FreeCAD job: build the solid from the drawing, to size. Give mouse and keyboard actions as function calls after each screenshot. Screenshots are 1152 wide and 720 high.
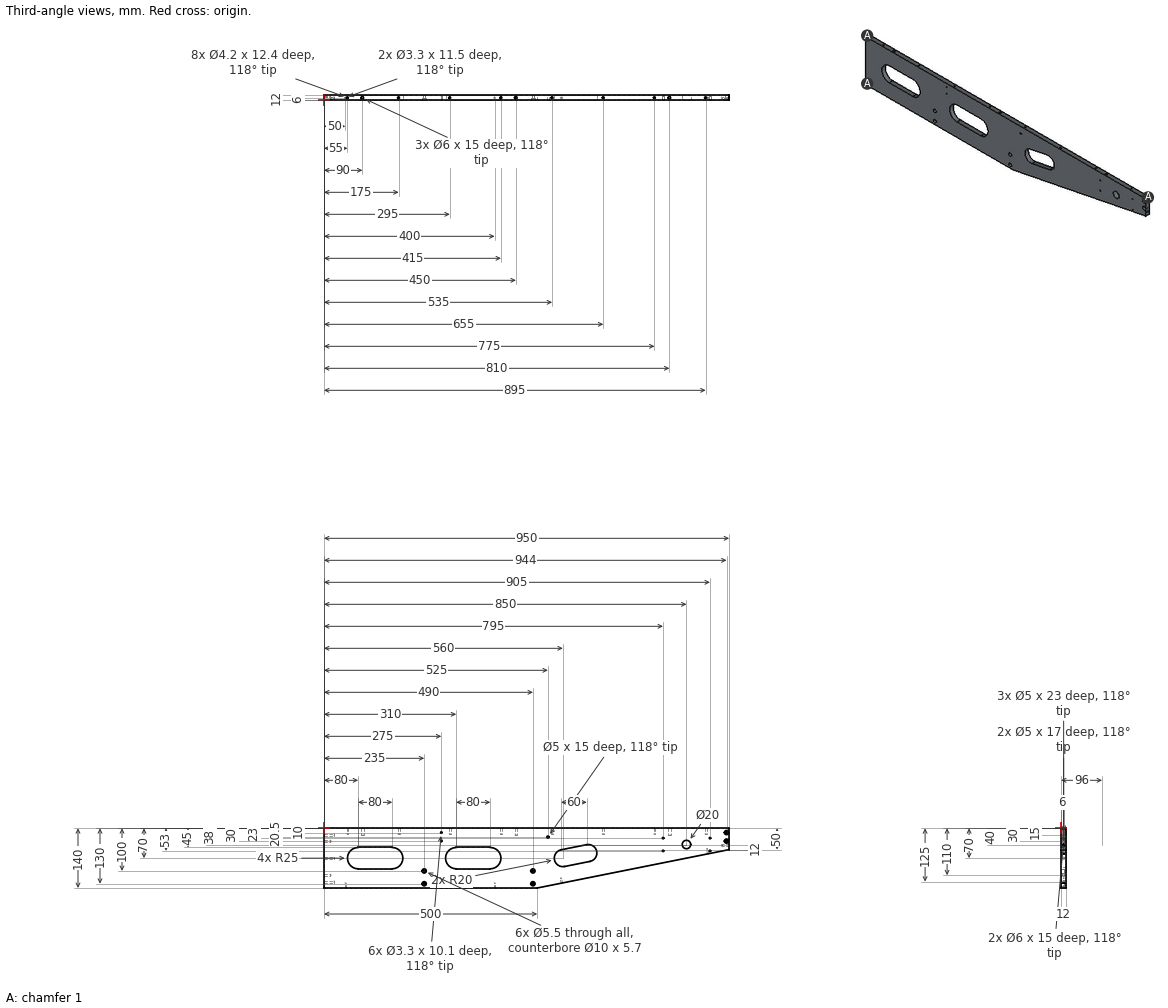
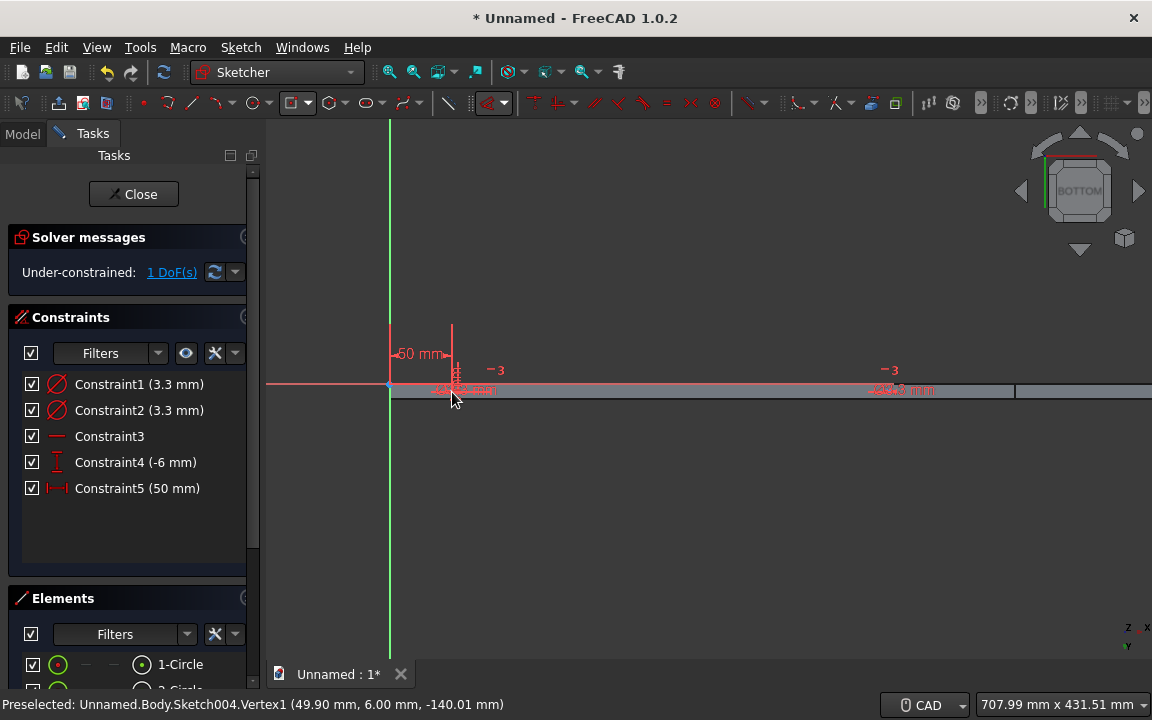
click(890, 392)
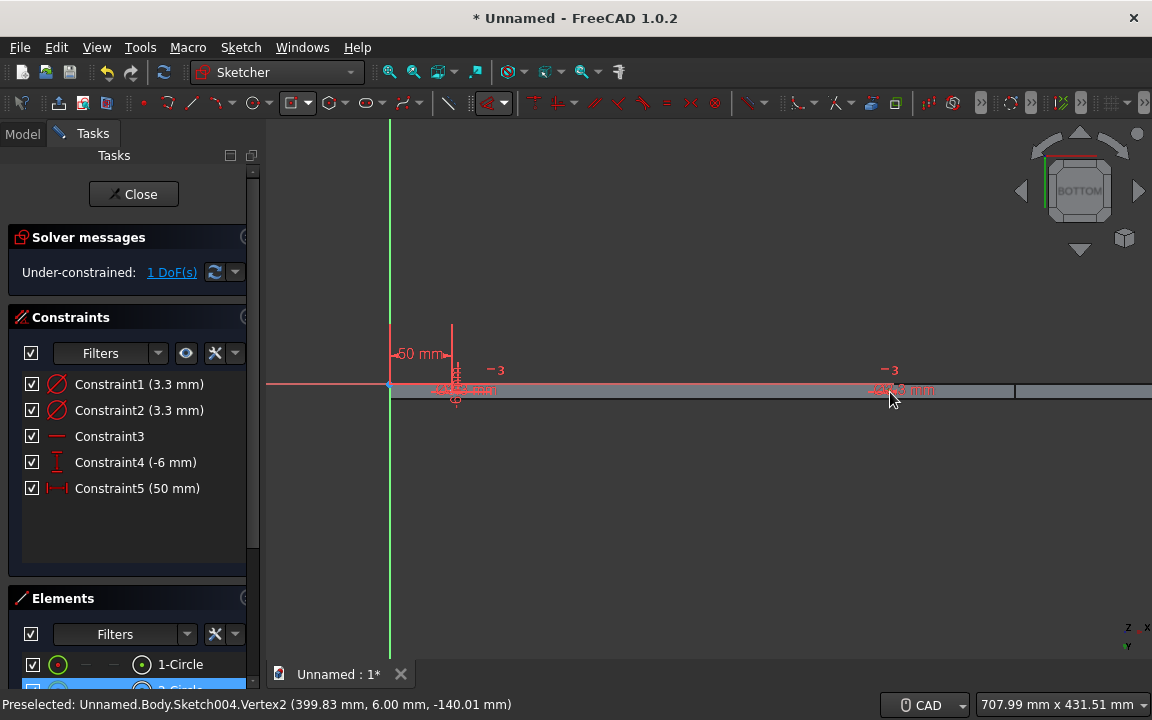
key(l)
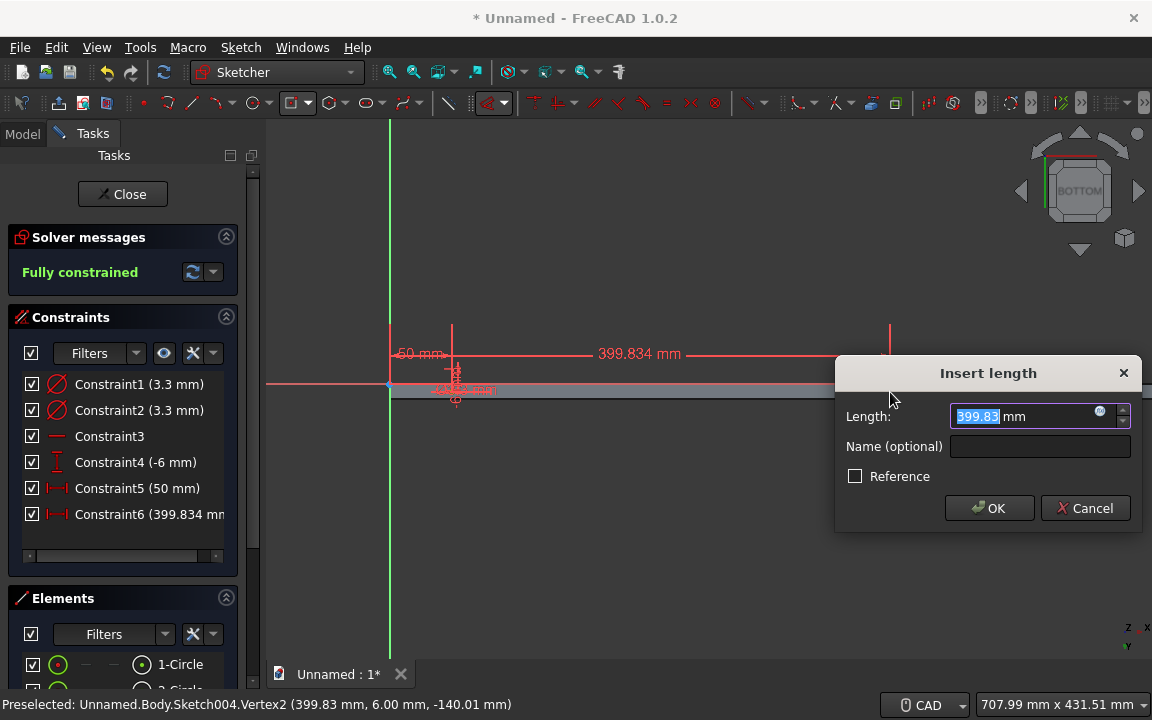
text(400)
key(Return)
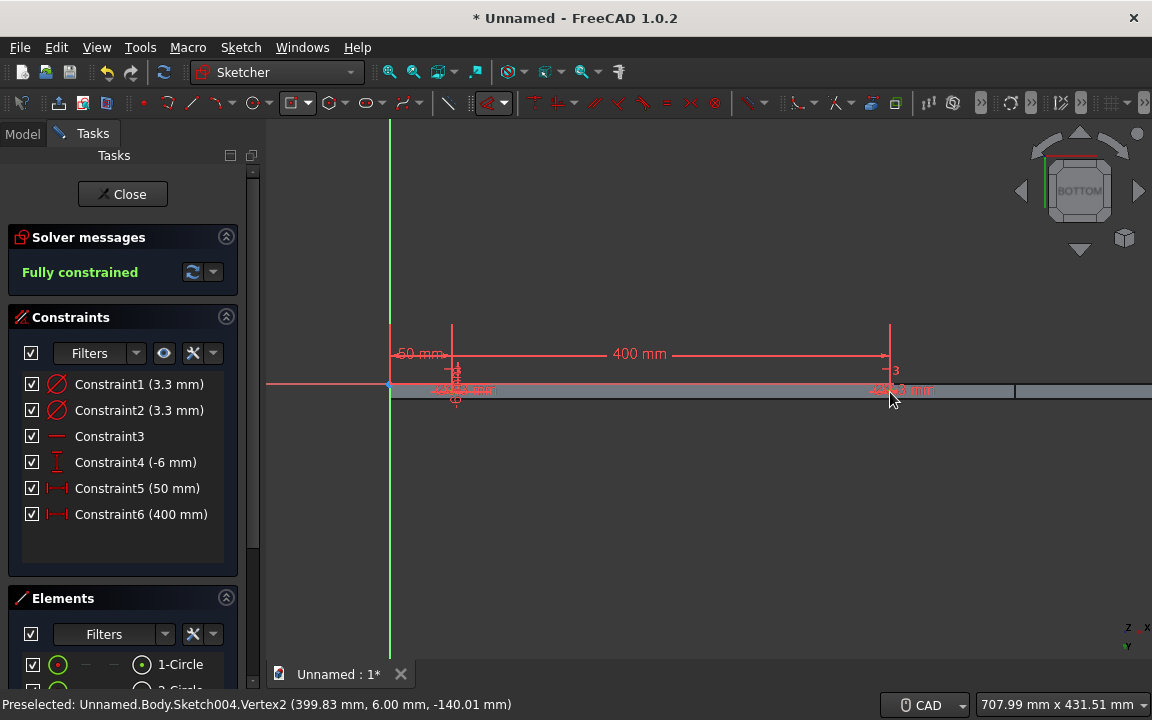
click(123, 194)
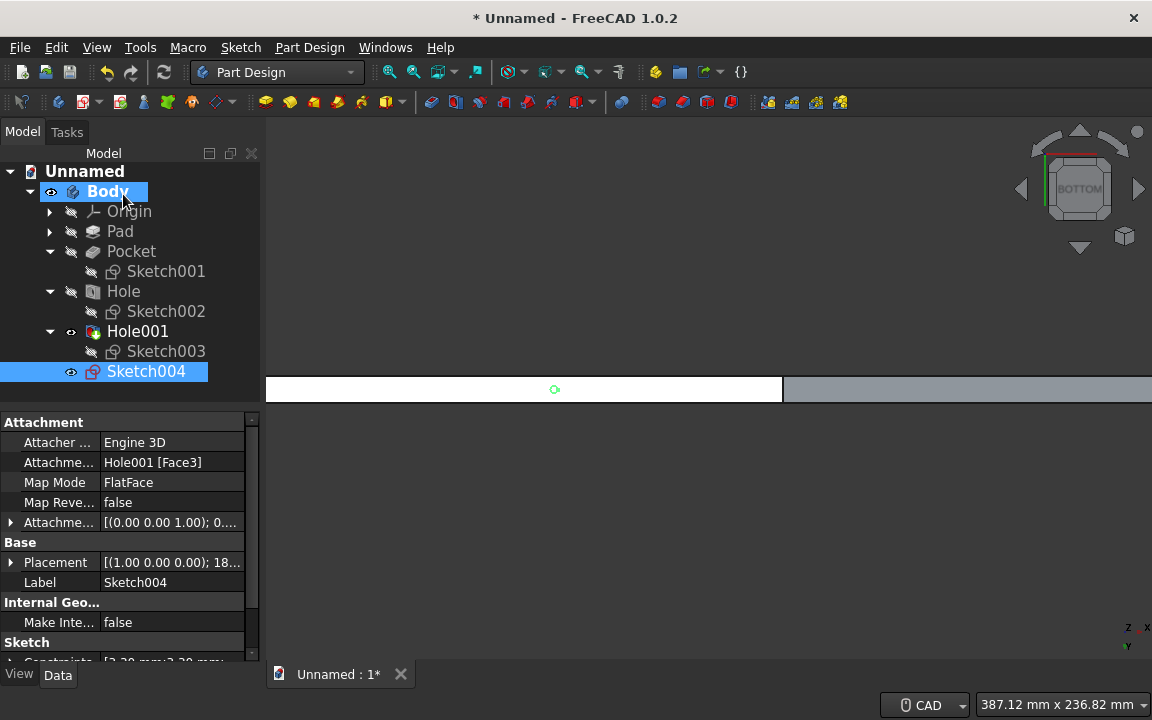
click(456, 102)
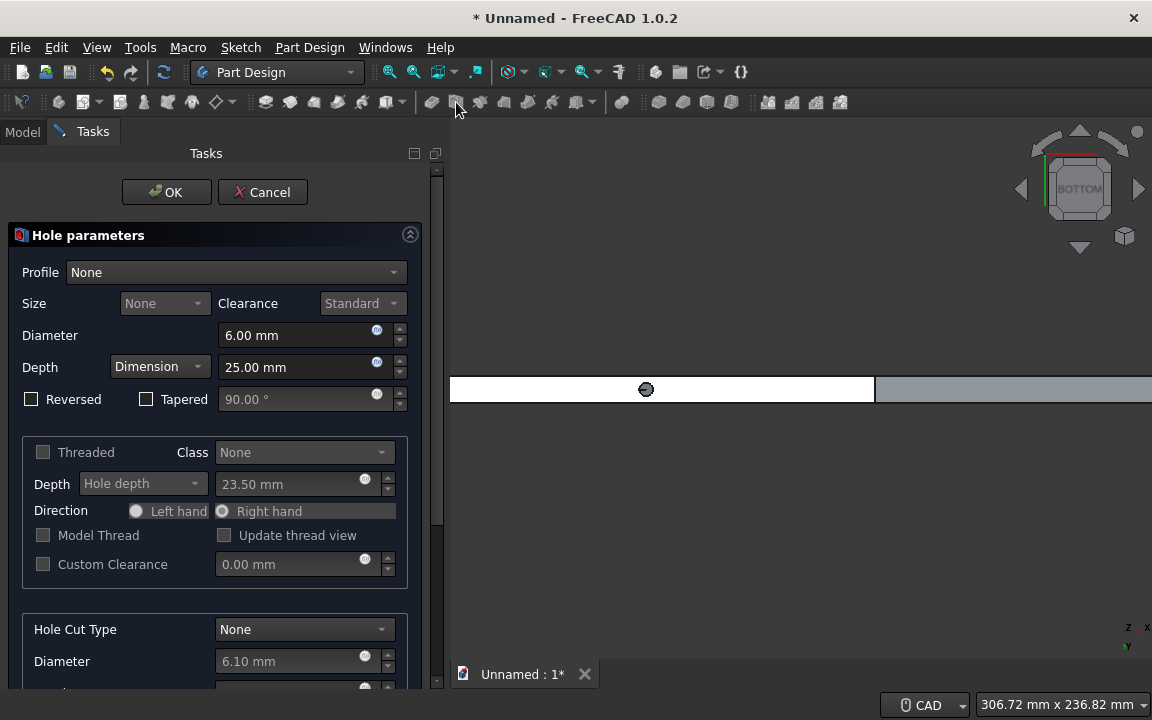
triple_click(305, 335)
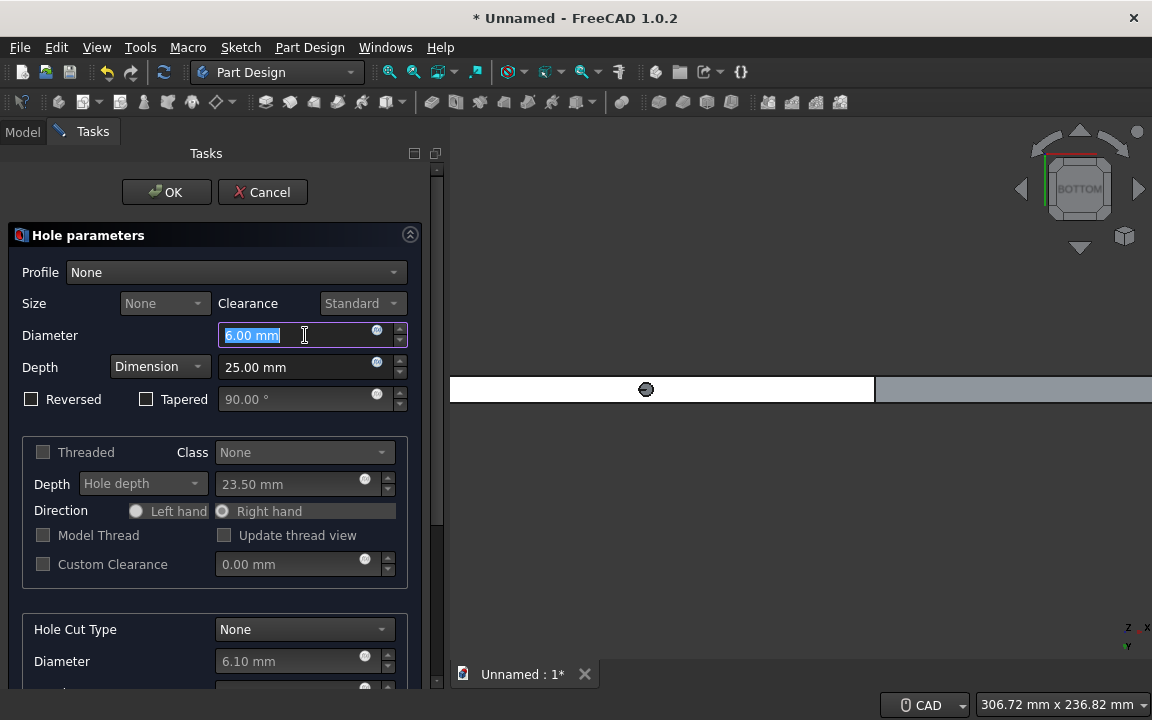
text(3.3)
key(Tab)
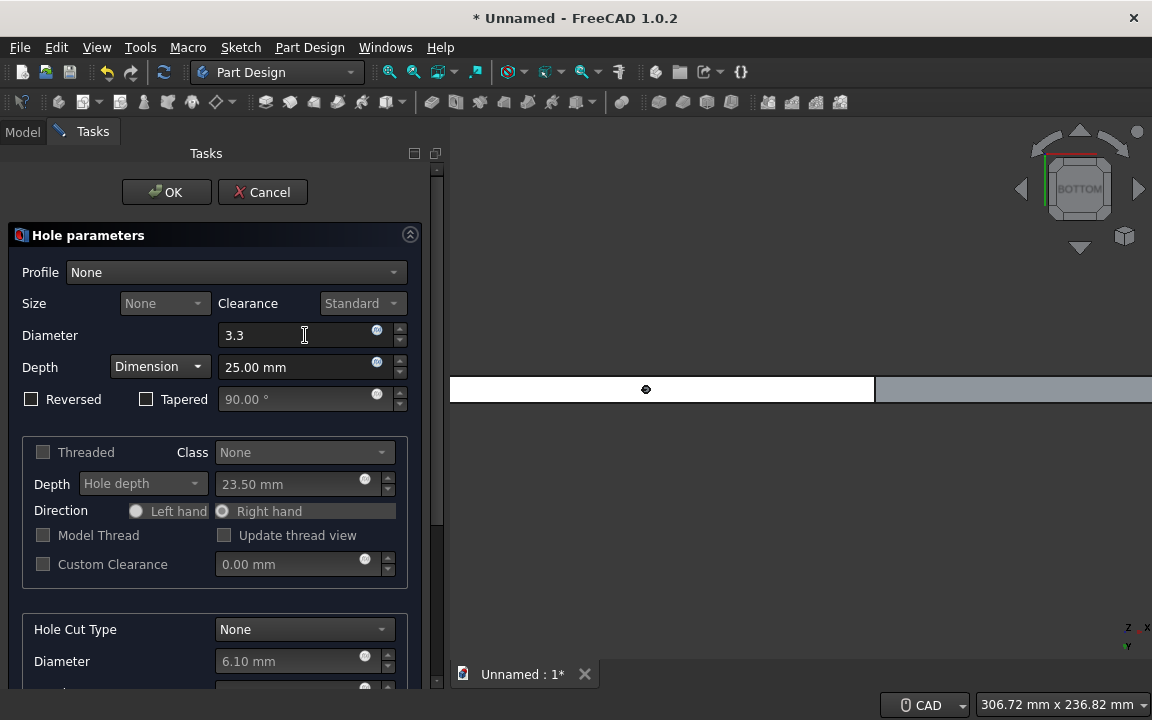
triple_click(305, 367)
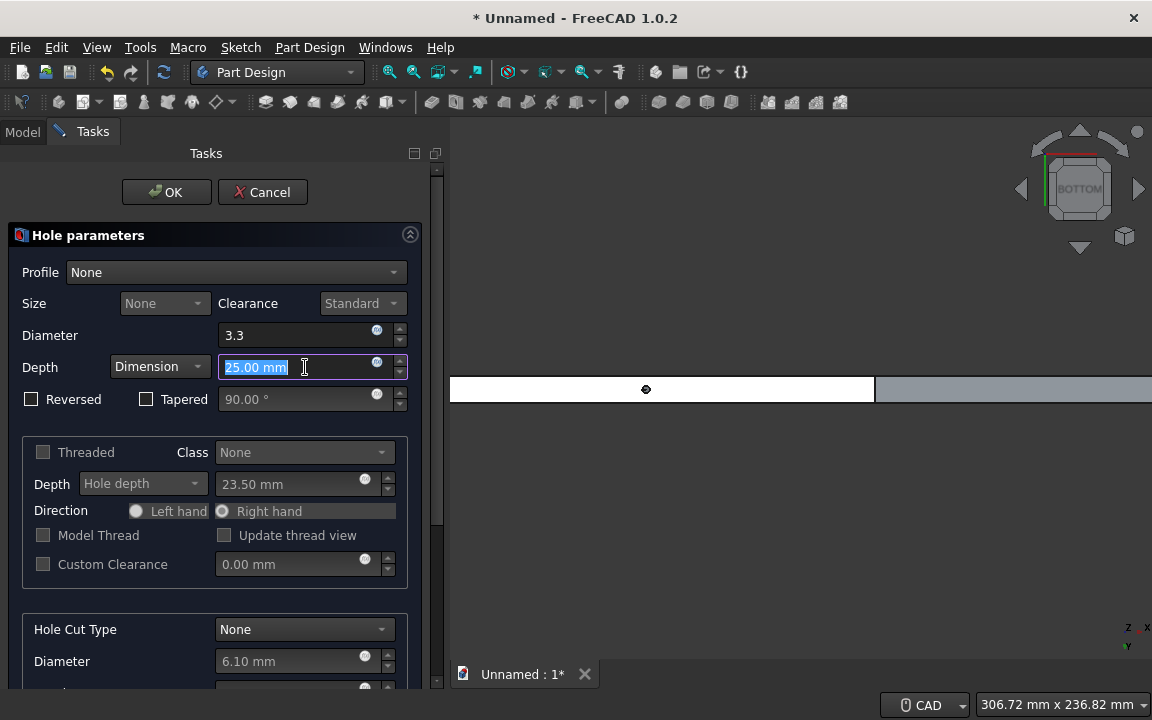
text(11.5)
key(Tab)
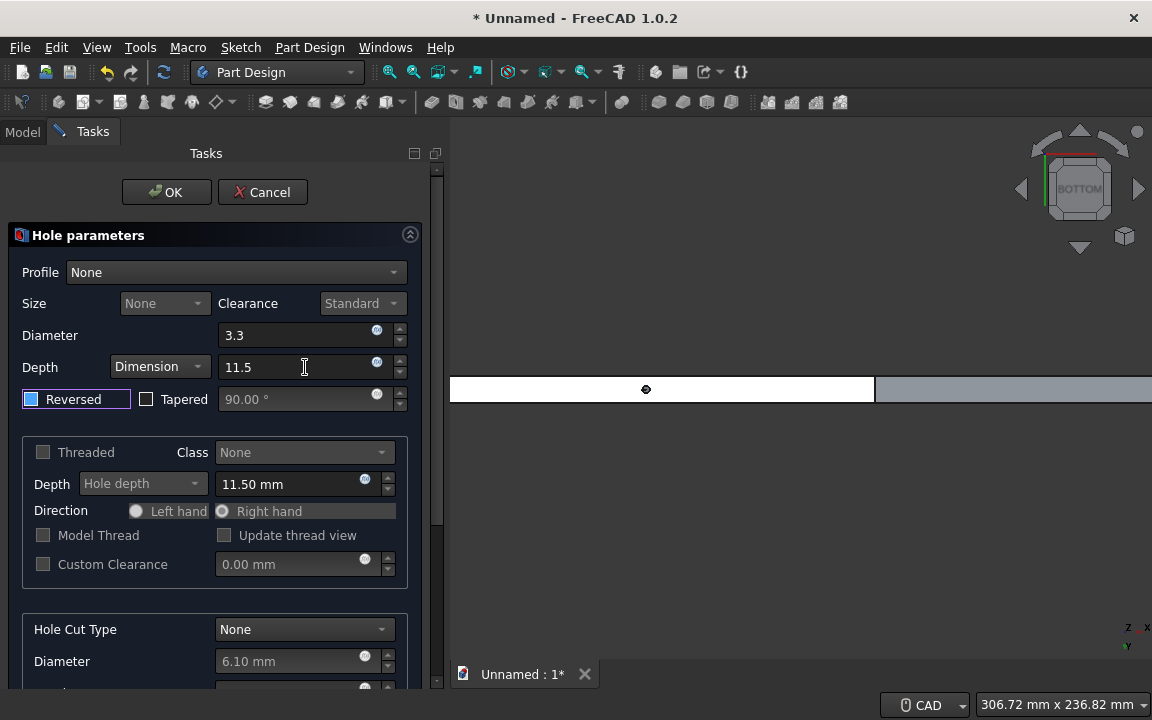
click(167, 192)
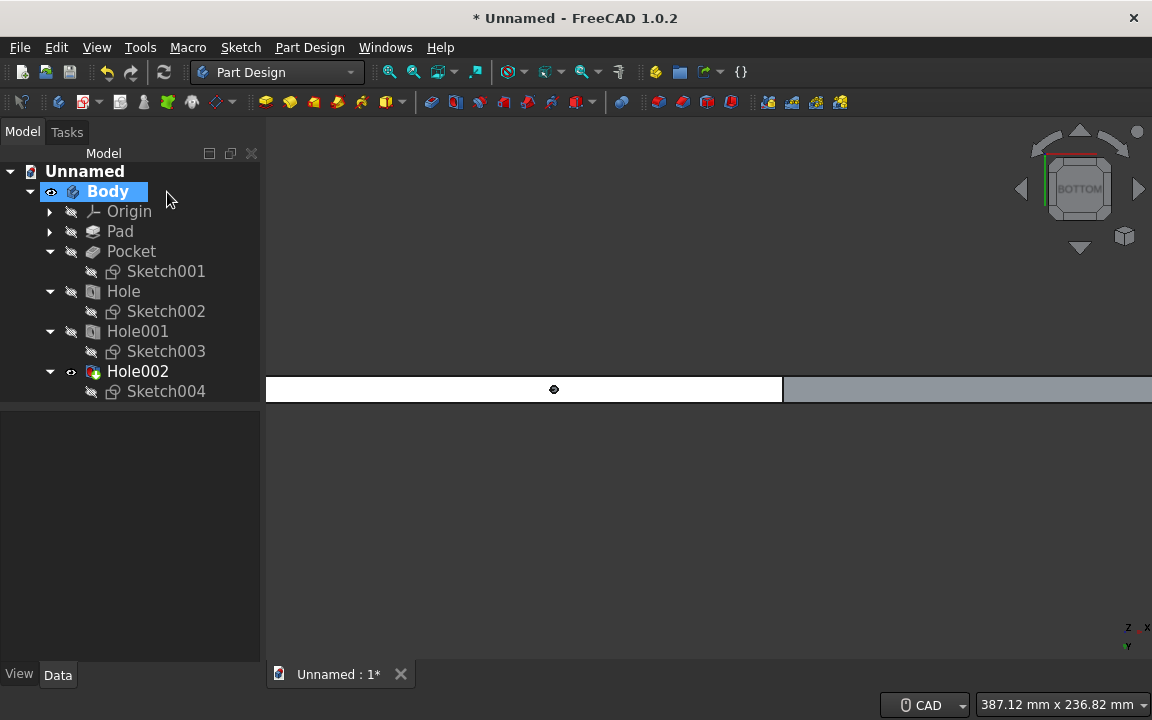
key(v)
key(f)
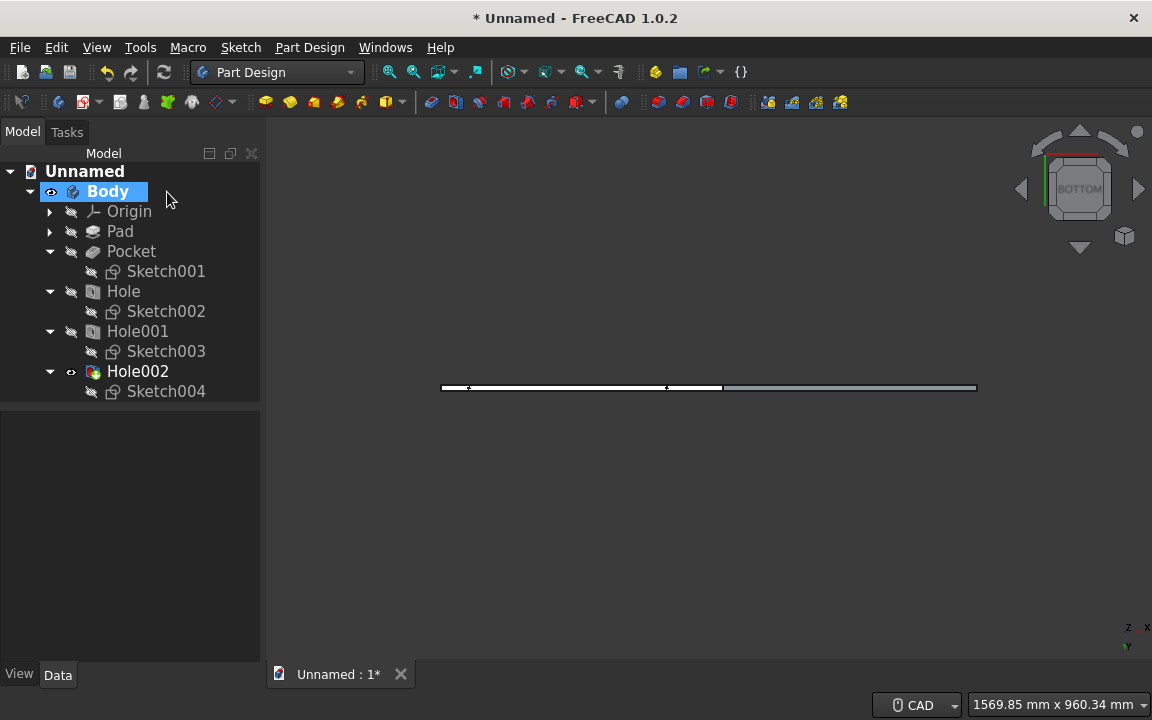
scroll(850, 387, up, 7)